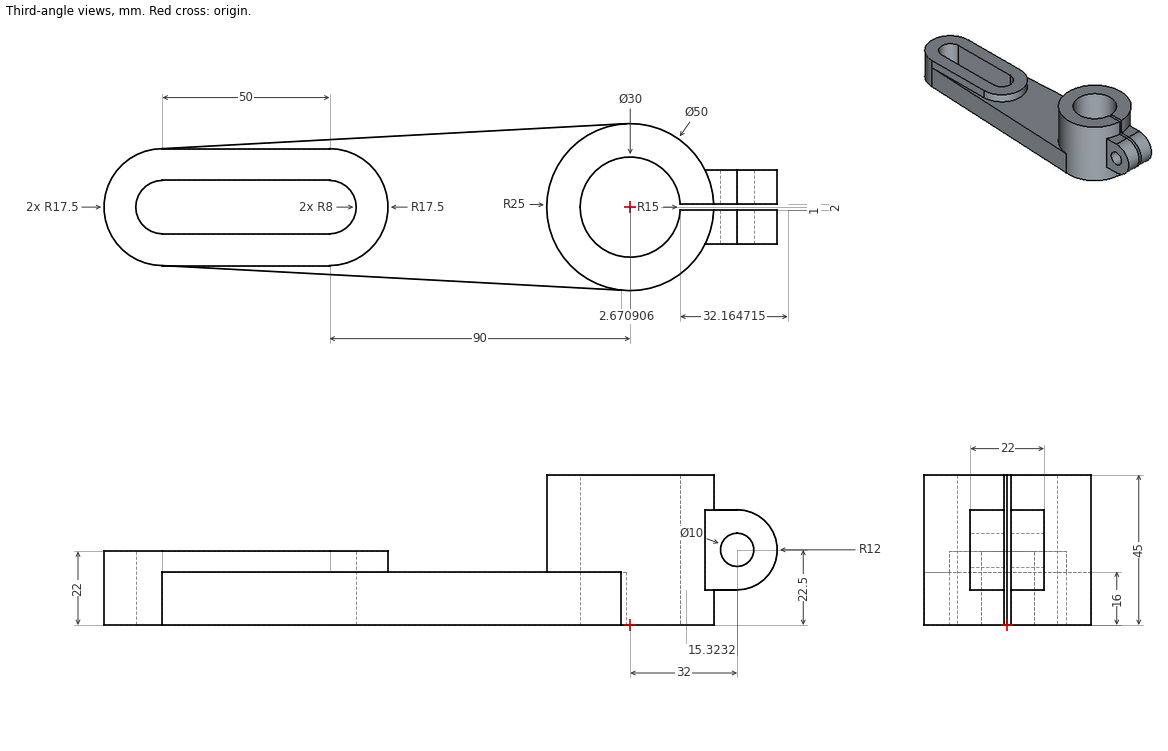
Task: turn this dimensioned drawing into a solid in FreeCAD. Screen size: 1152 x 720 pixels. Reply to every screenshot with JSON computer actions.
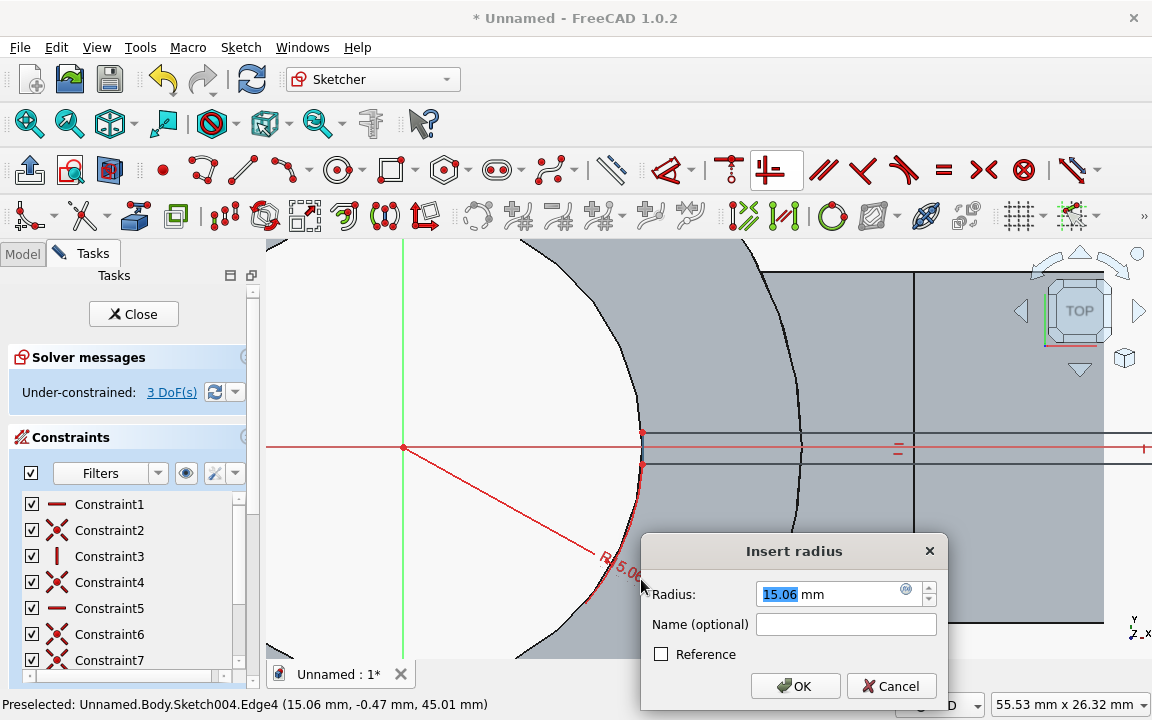
{"action": "type", "text": "15"}
{"action": "key", "text": "Return"}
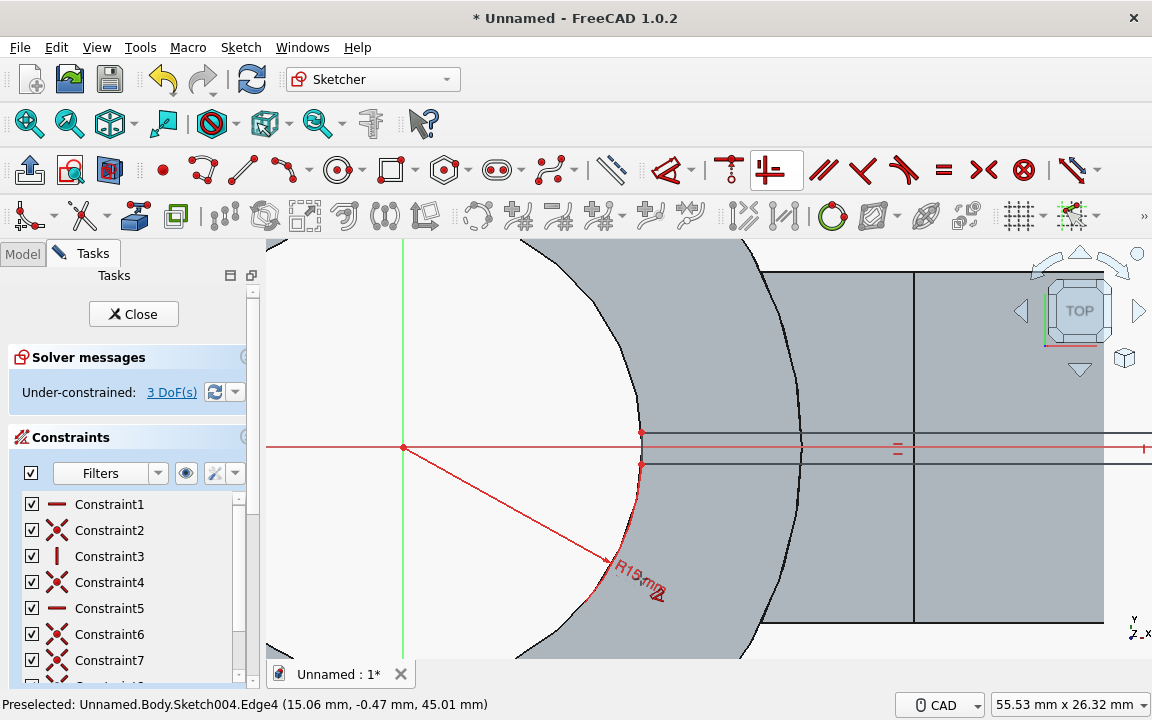
{"action": "scroll", "coordinate": [359, 452], "scroll_direction": "down", "scroll_amount": 2}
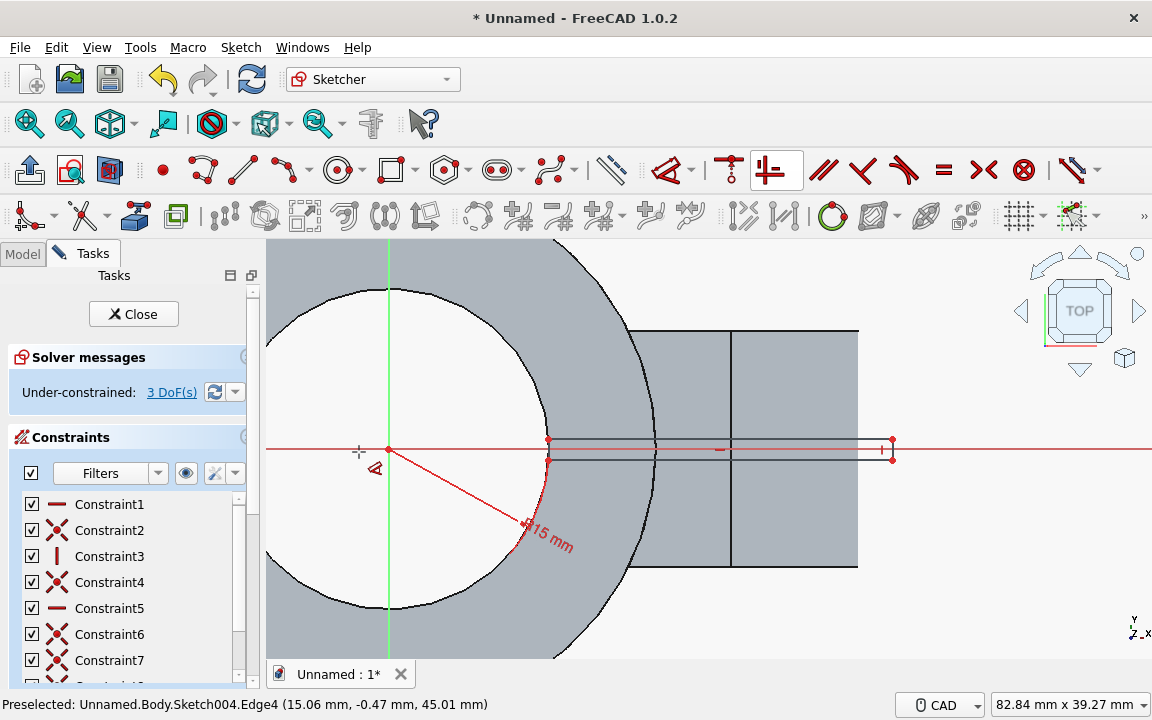
{"action": "scroll", "coordinate": [893, 448], "scroll_direction": "up", "scroll_amount": 4}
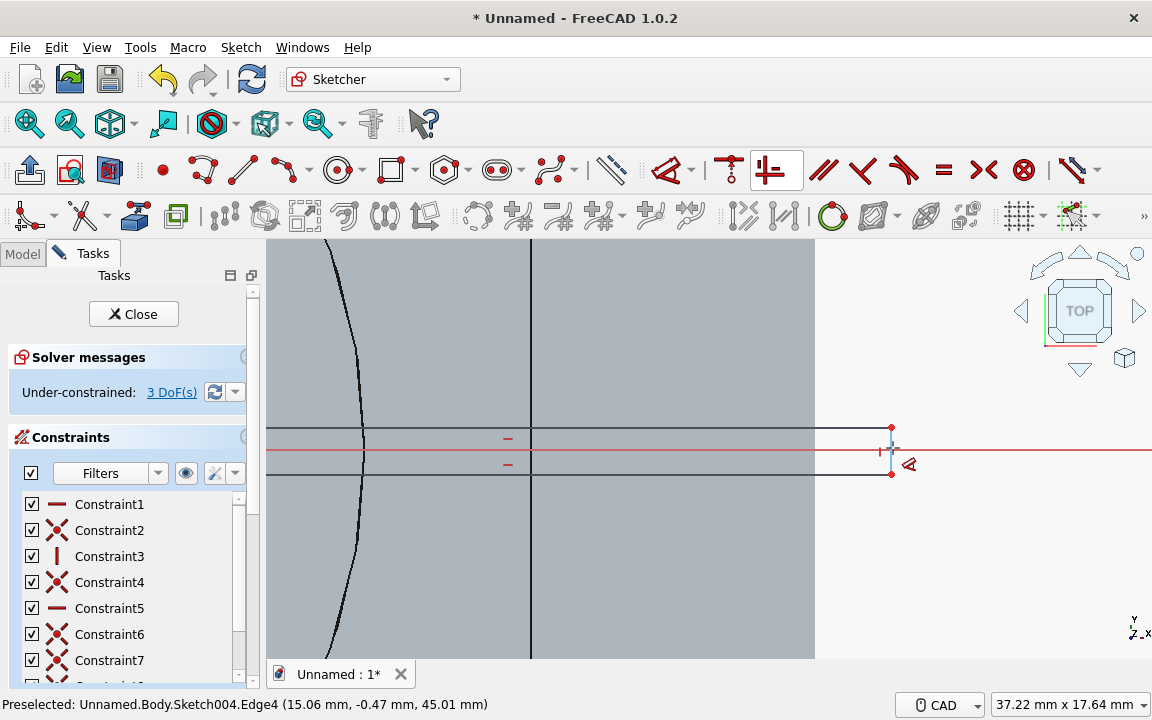
{"action": "left_click", "coordinate": [891, 447]}
{"action": "left_click", "coordinate": [925, 435]}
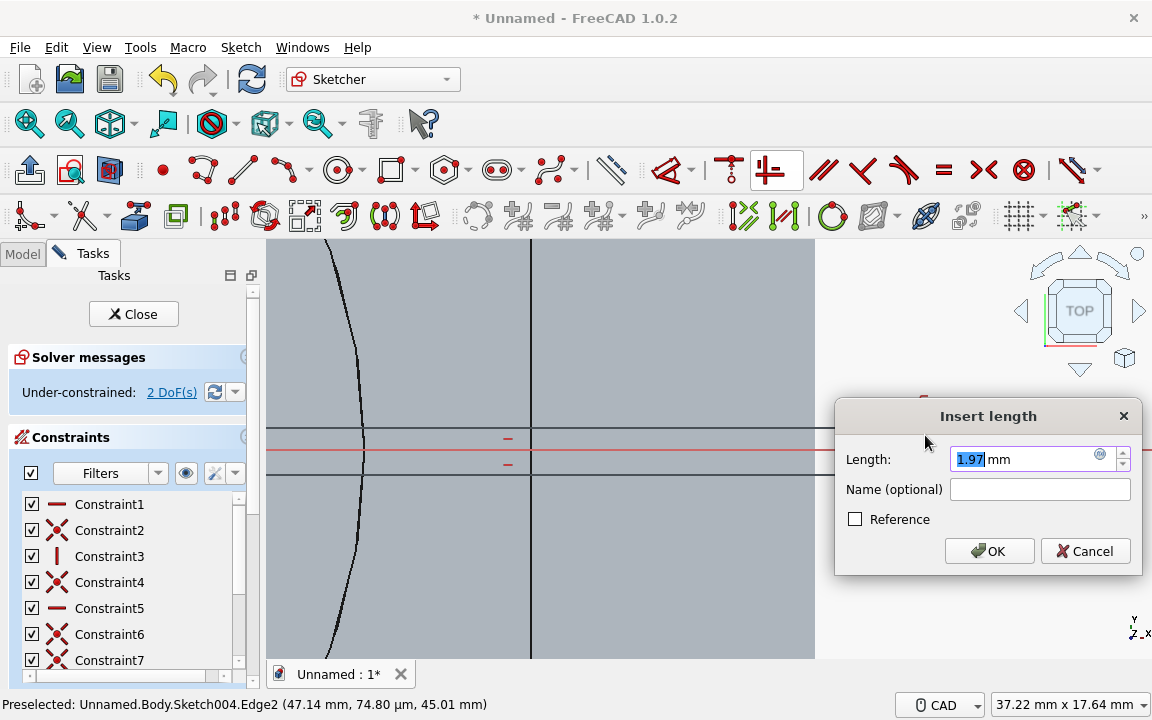
{"action": "type", "text": "2"}
{"action": "key", "text": "Return"}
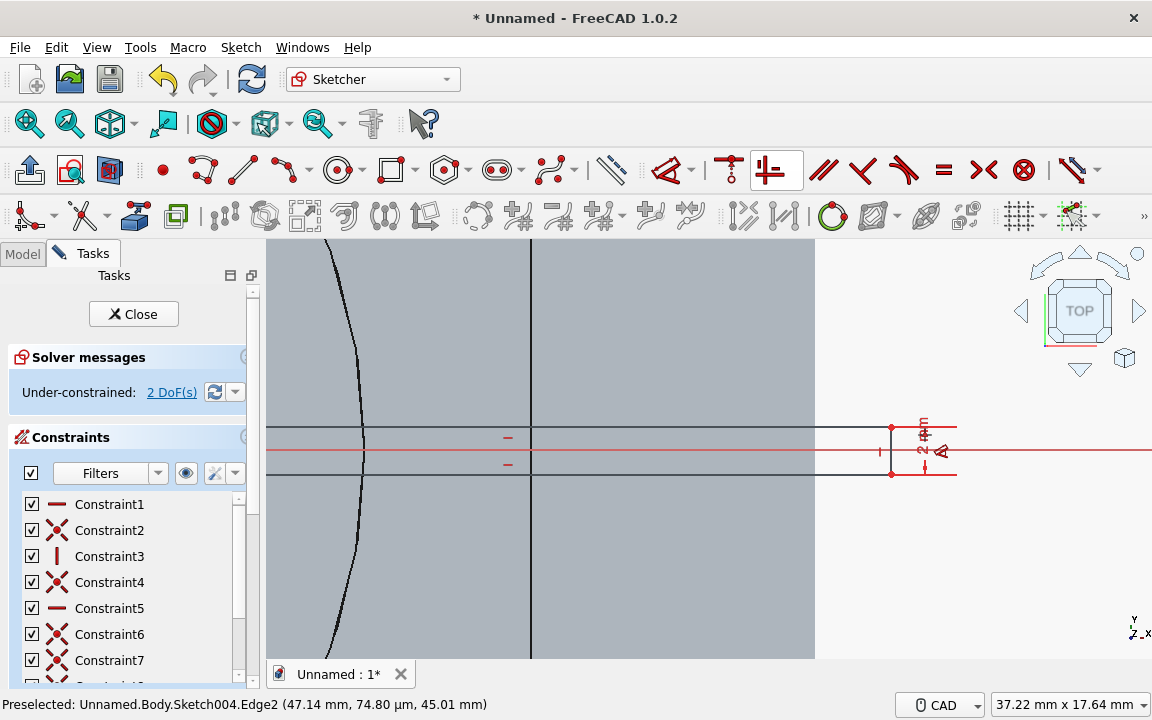
{"action": "scroll", "coordinate": [894, 448], "scroll_direction": "down", "scroll_amount": 4}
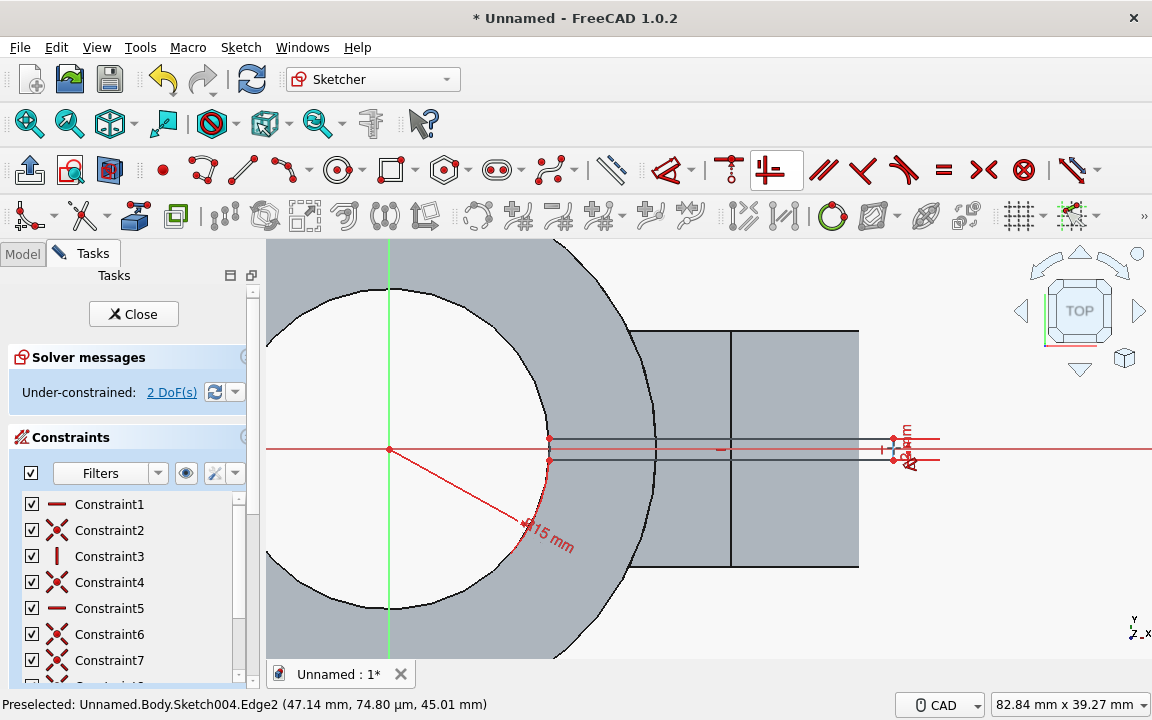
{"action": "scroll", "coordinate": [549, 460], "scroll_direction": "up", "scroll_amount": 7}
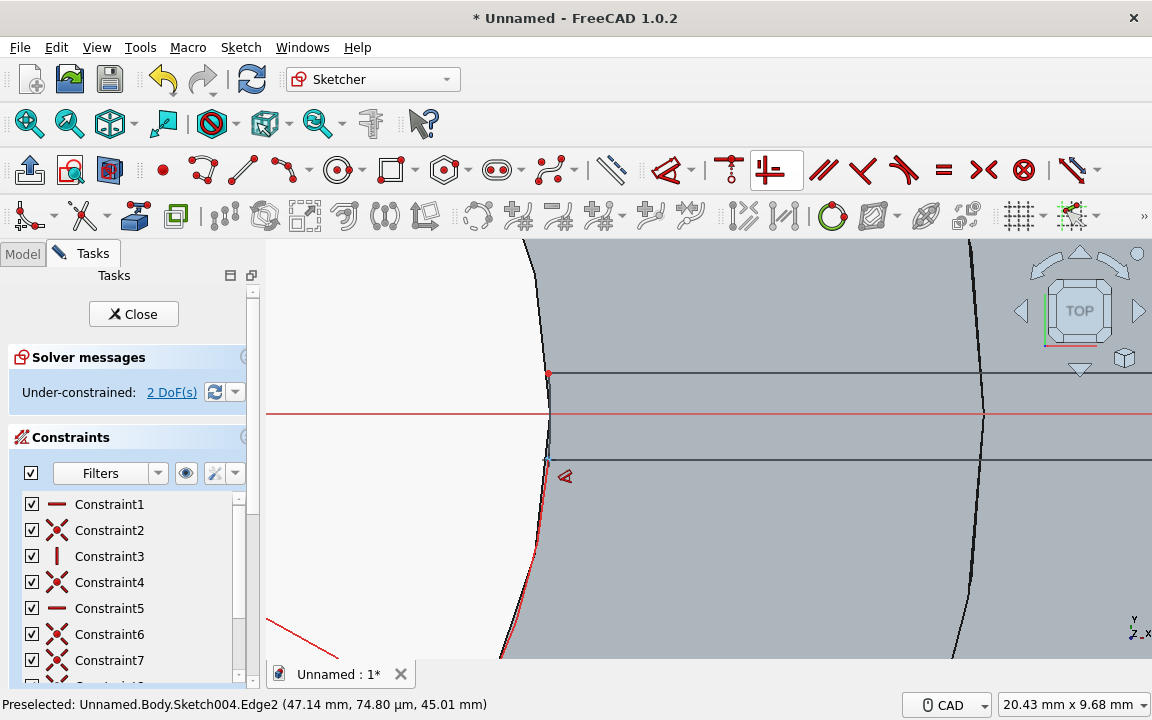
{"action": "left_click", "coordinate": [549, 460]}
{"action": "left_click", "coordinate": [583, 437]}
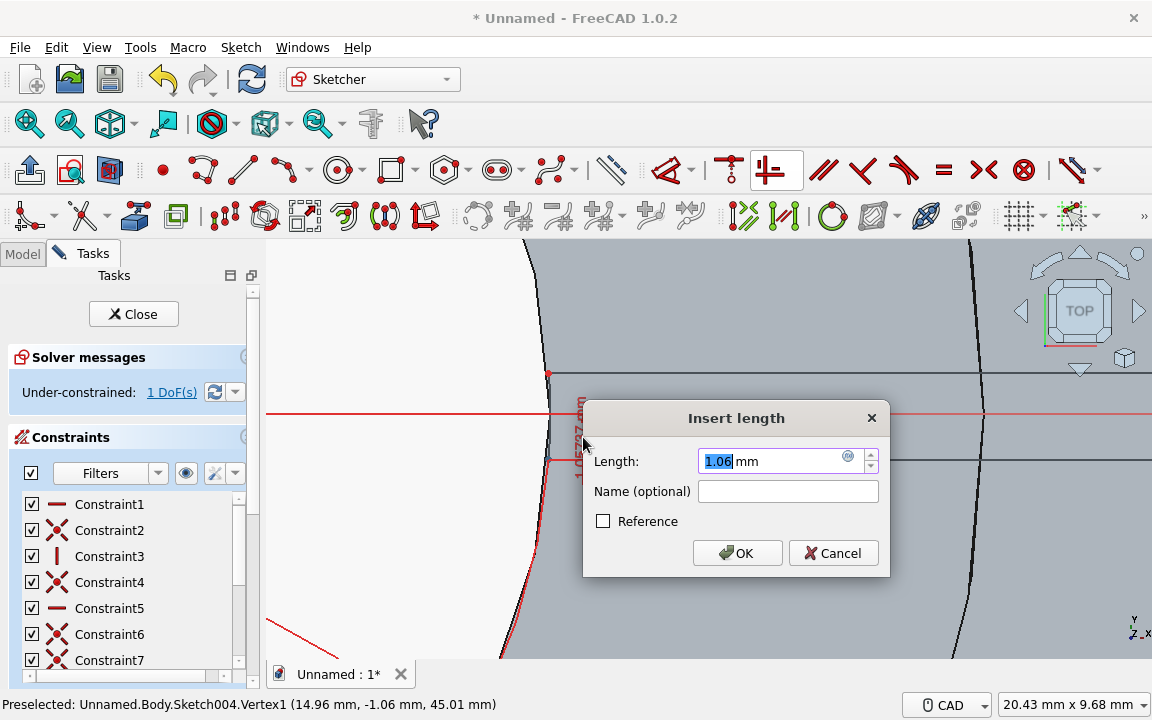
{"action": "type", "text": "1"}
{"action": "key", "text": "Return"}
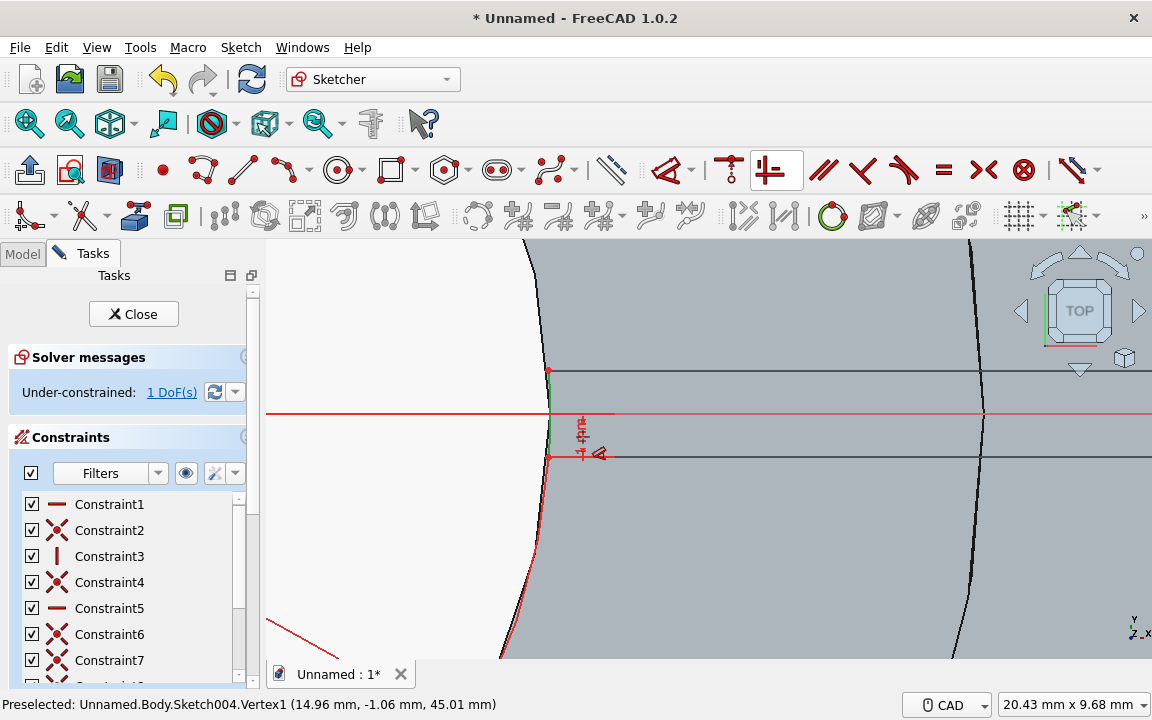
{"action": "scroll", "coordinate": [548, 460], "scroll_direction": "down", "scroll_amount": 7}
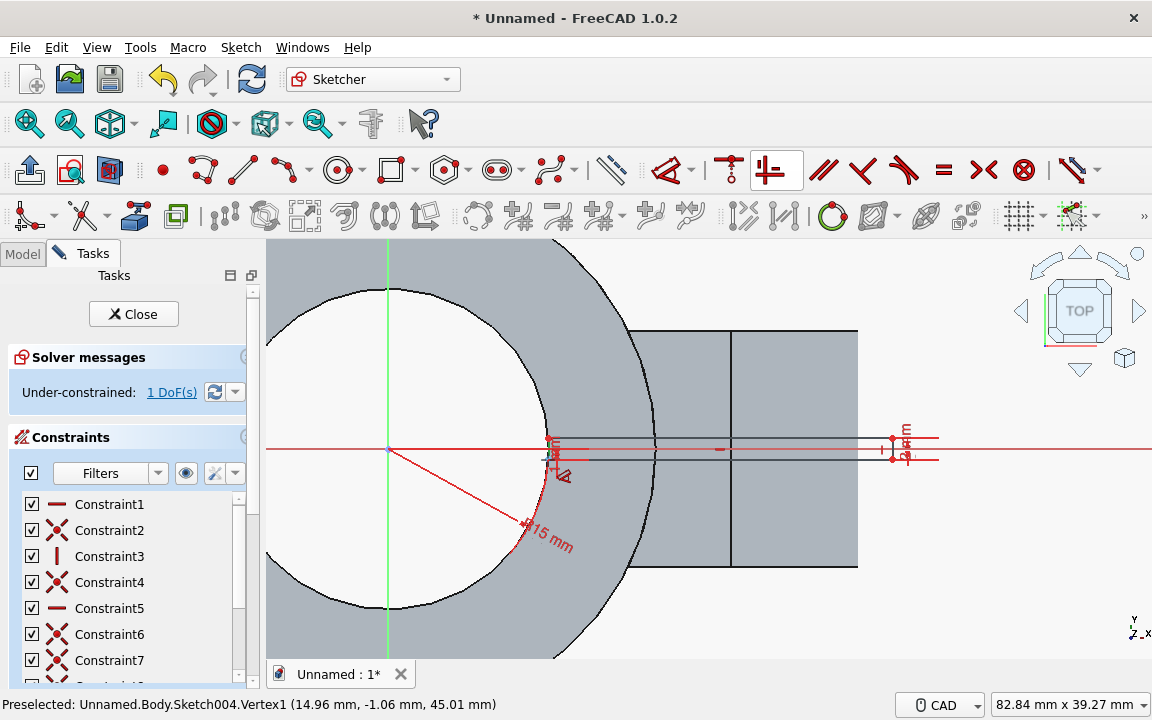
{"action": "scroll", "coordinate": [652, 460], "scroll_direction": "up", "scroll_amount": 2}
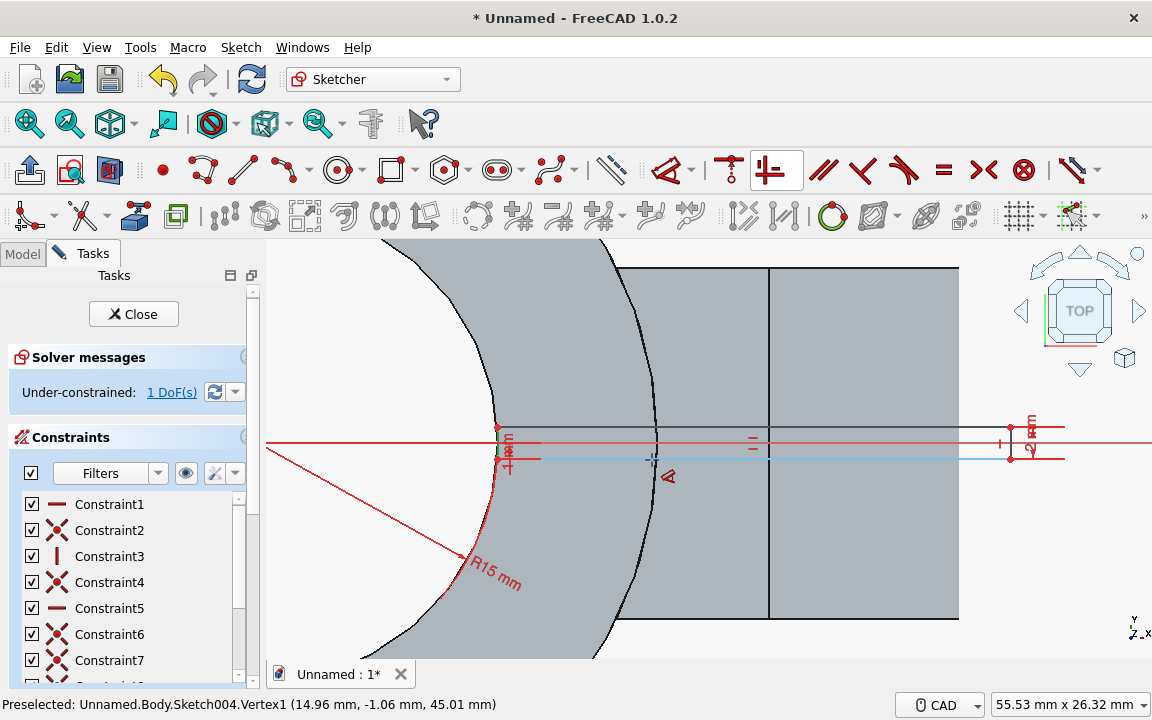
{"action": "left_click", "coordinate": [651, 459]}
{"action": "left_click", "coordinate": [742, 493]}